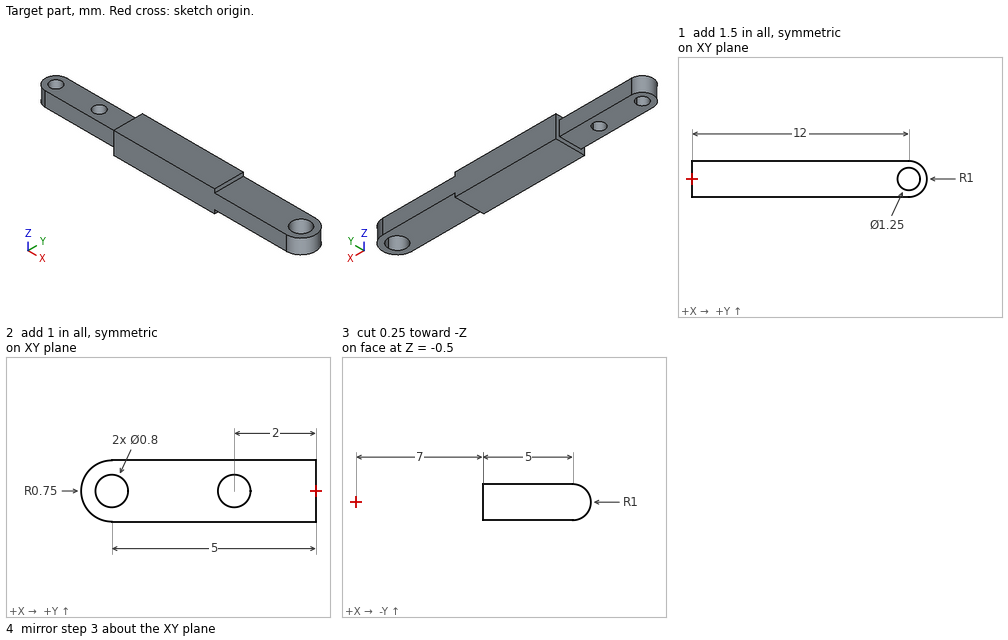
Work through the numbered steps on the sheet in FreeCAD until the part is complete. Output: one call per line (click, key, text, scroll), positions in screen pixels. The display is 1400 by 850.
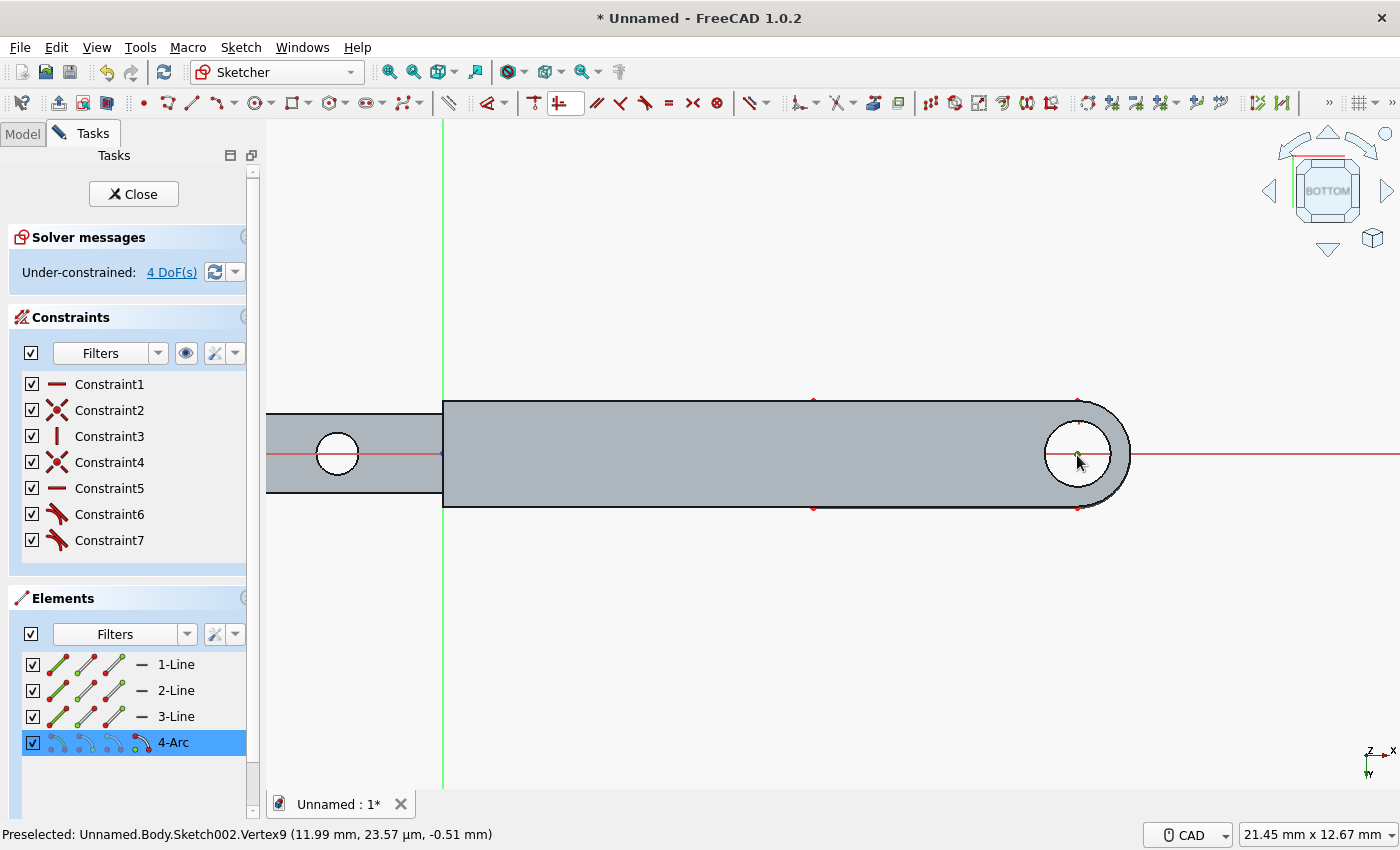
click(361, 454)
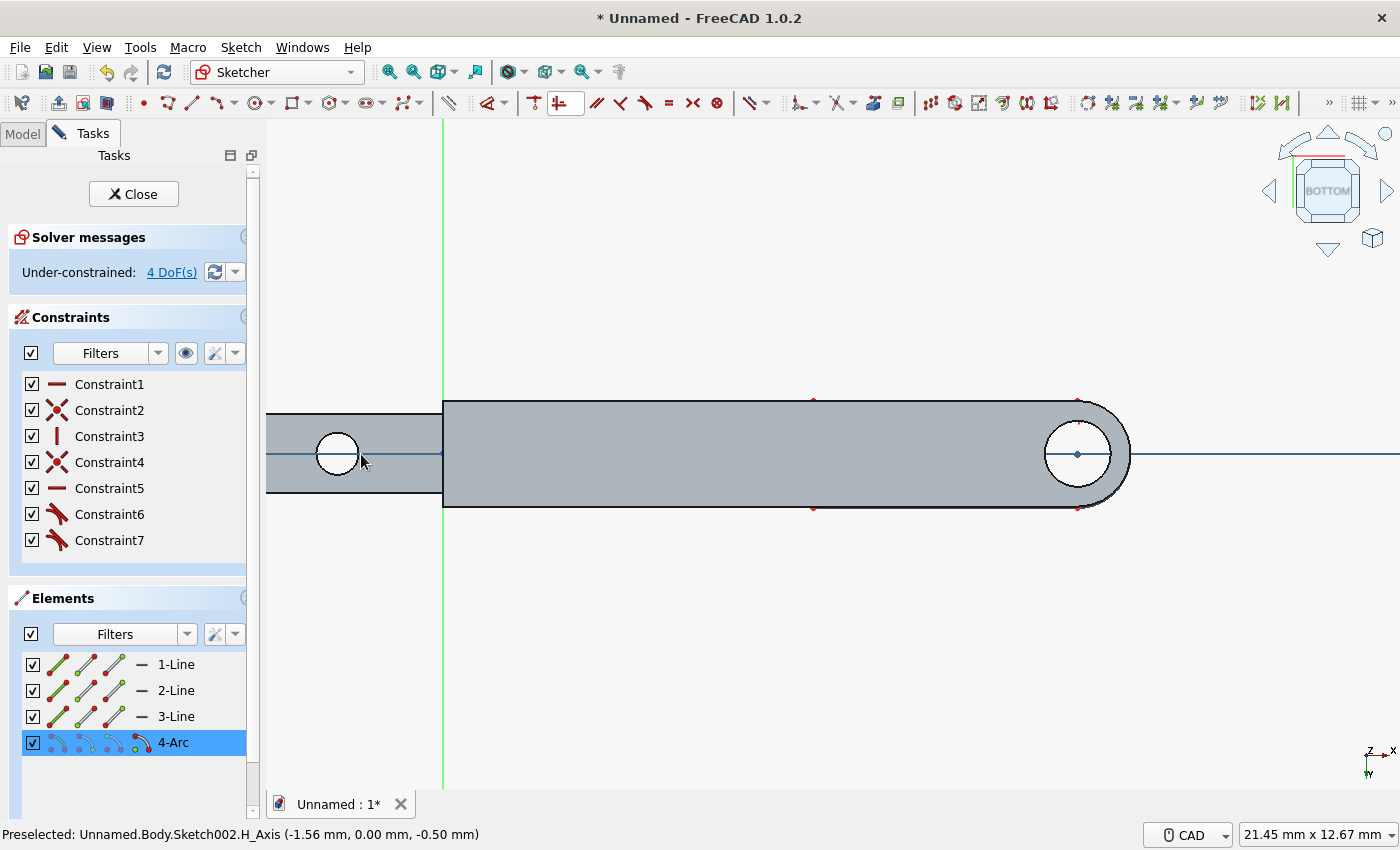
key(c)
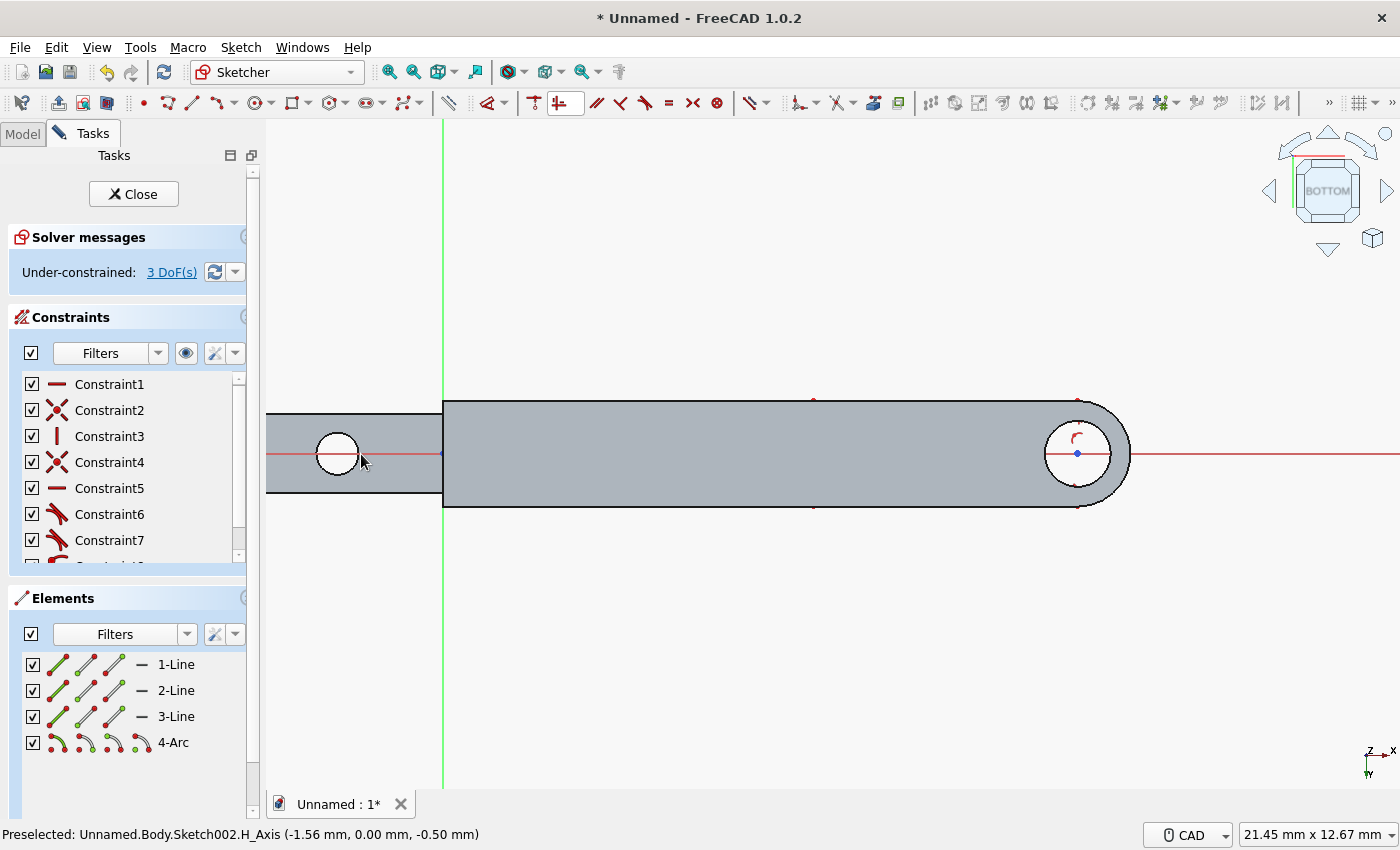
key(d)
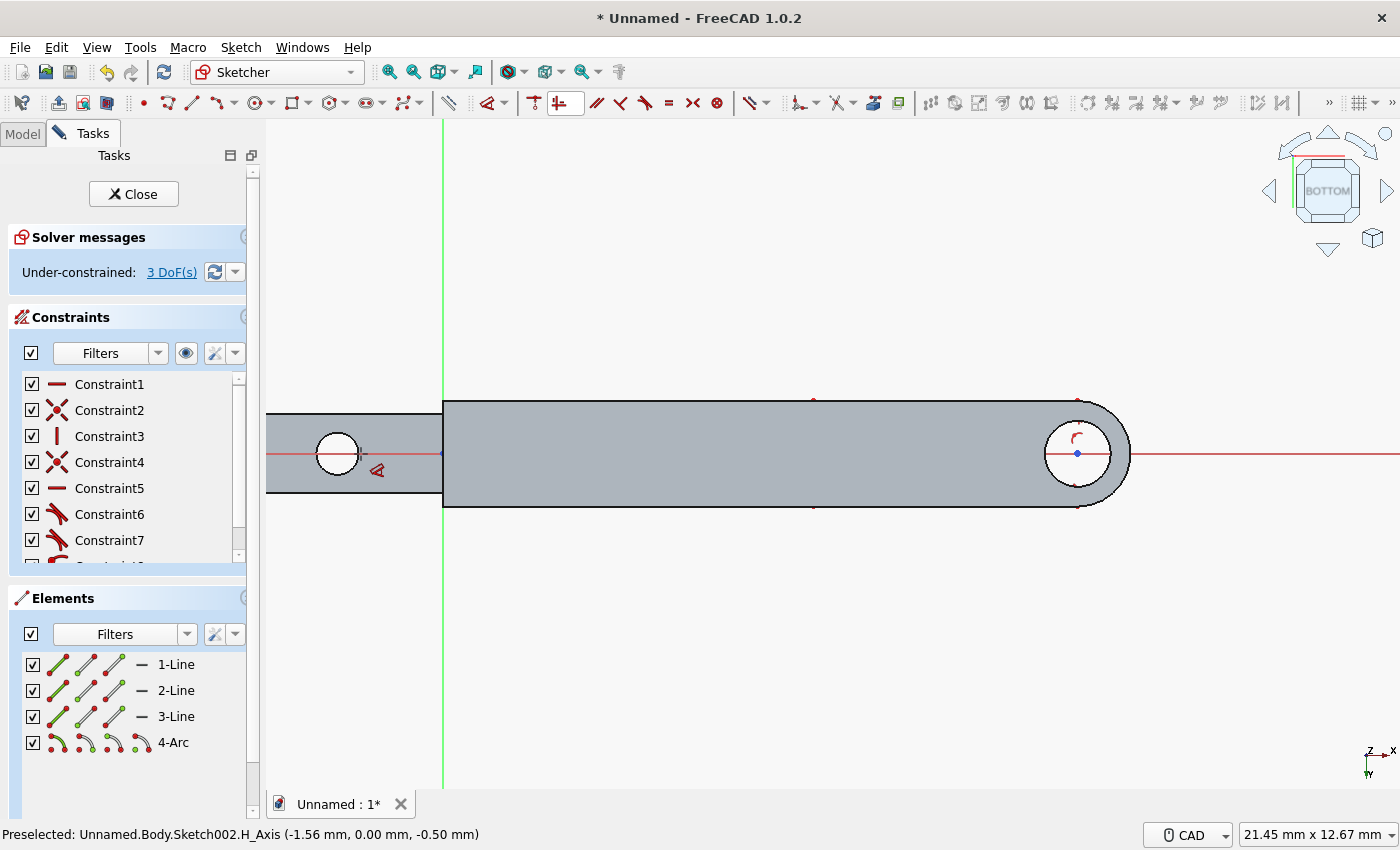
click(1119, 484)
click(1145, 503)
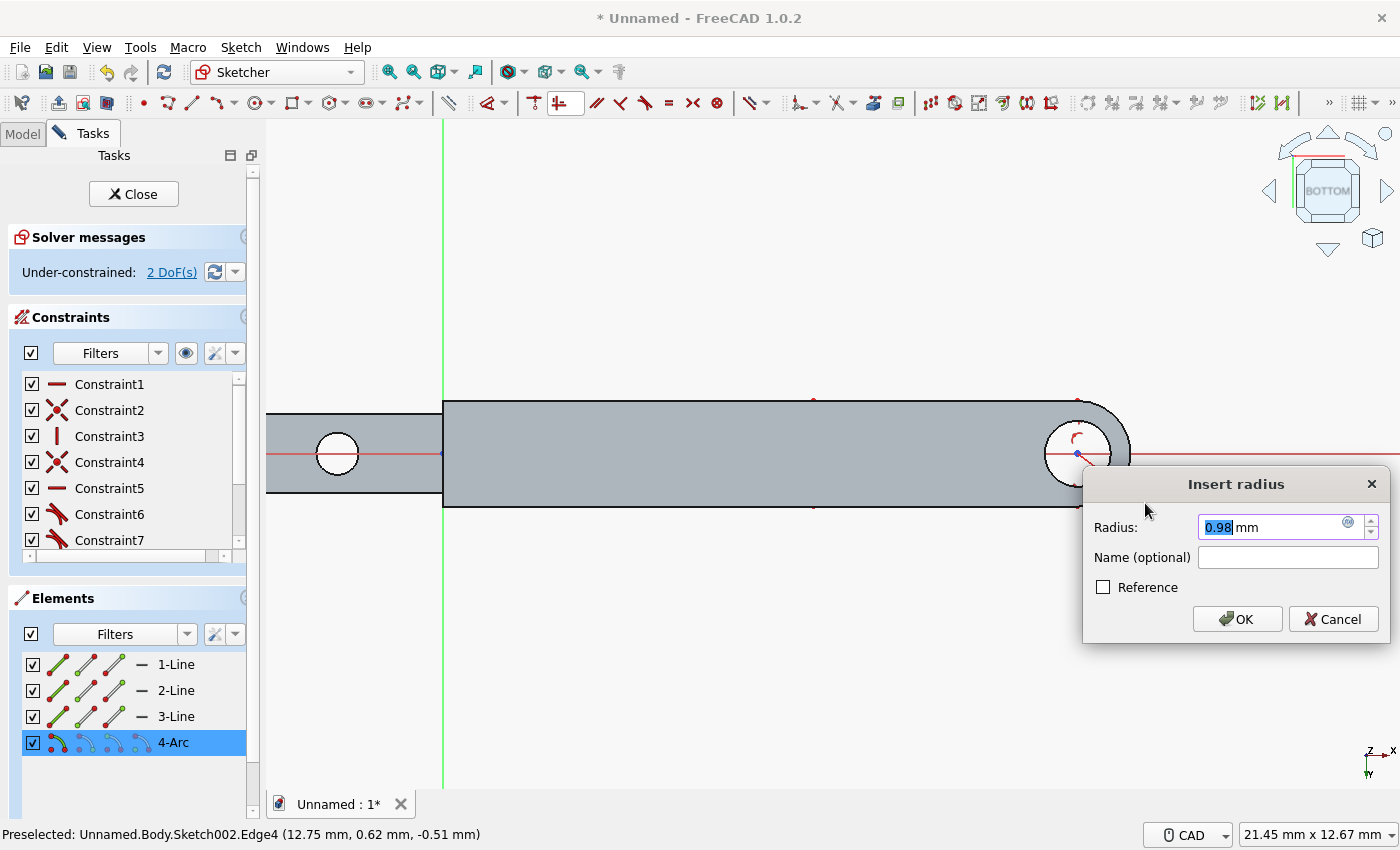
text(1)
key(Return)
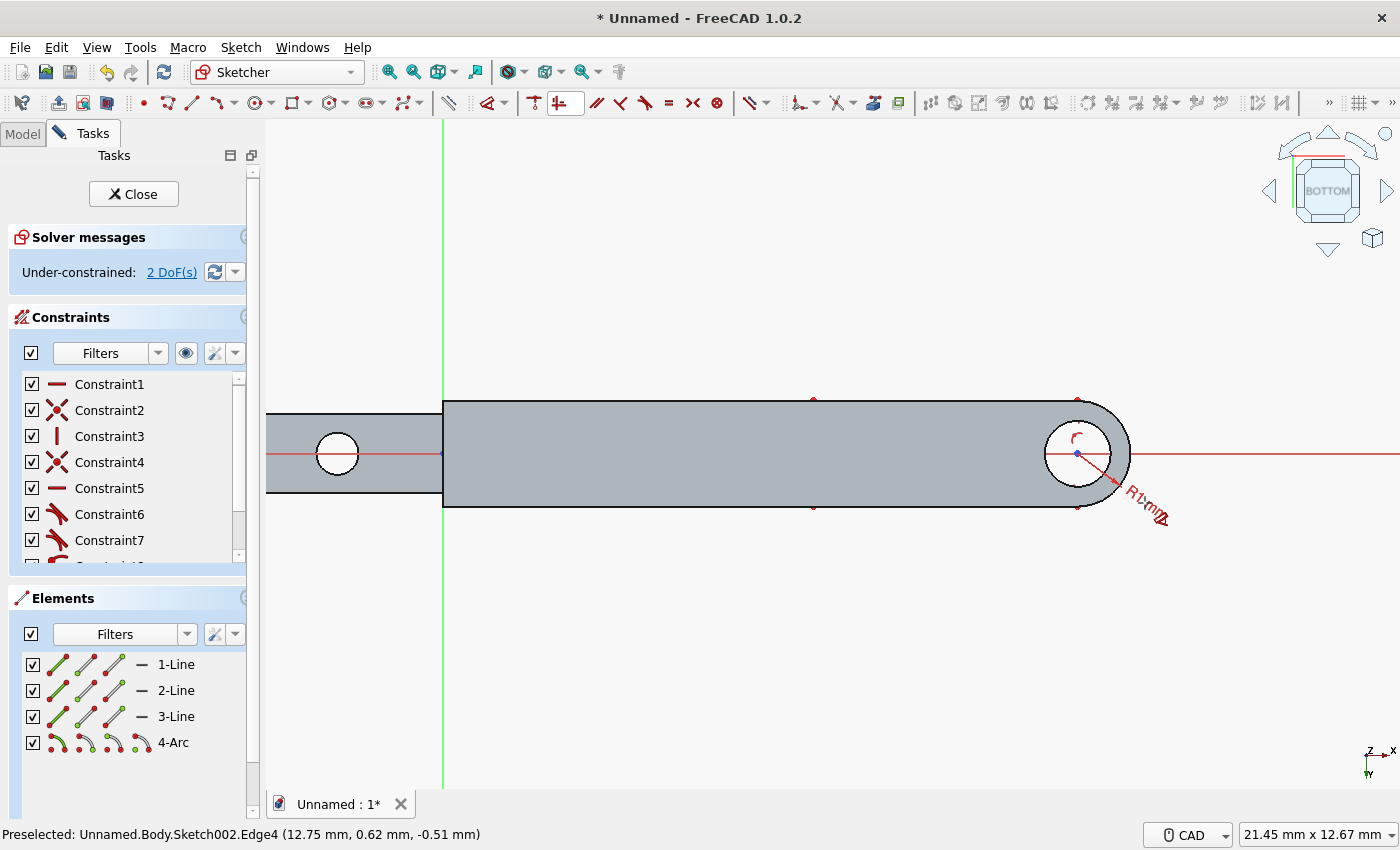
click(998, 401)
click(945, 367)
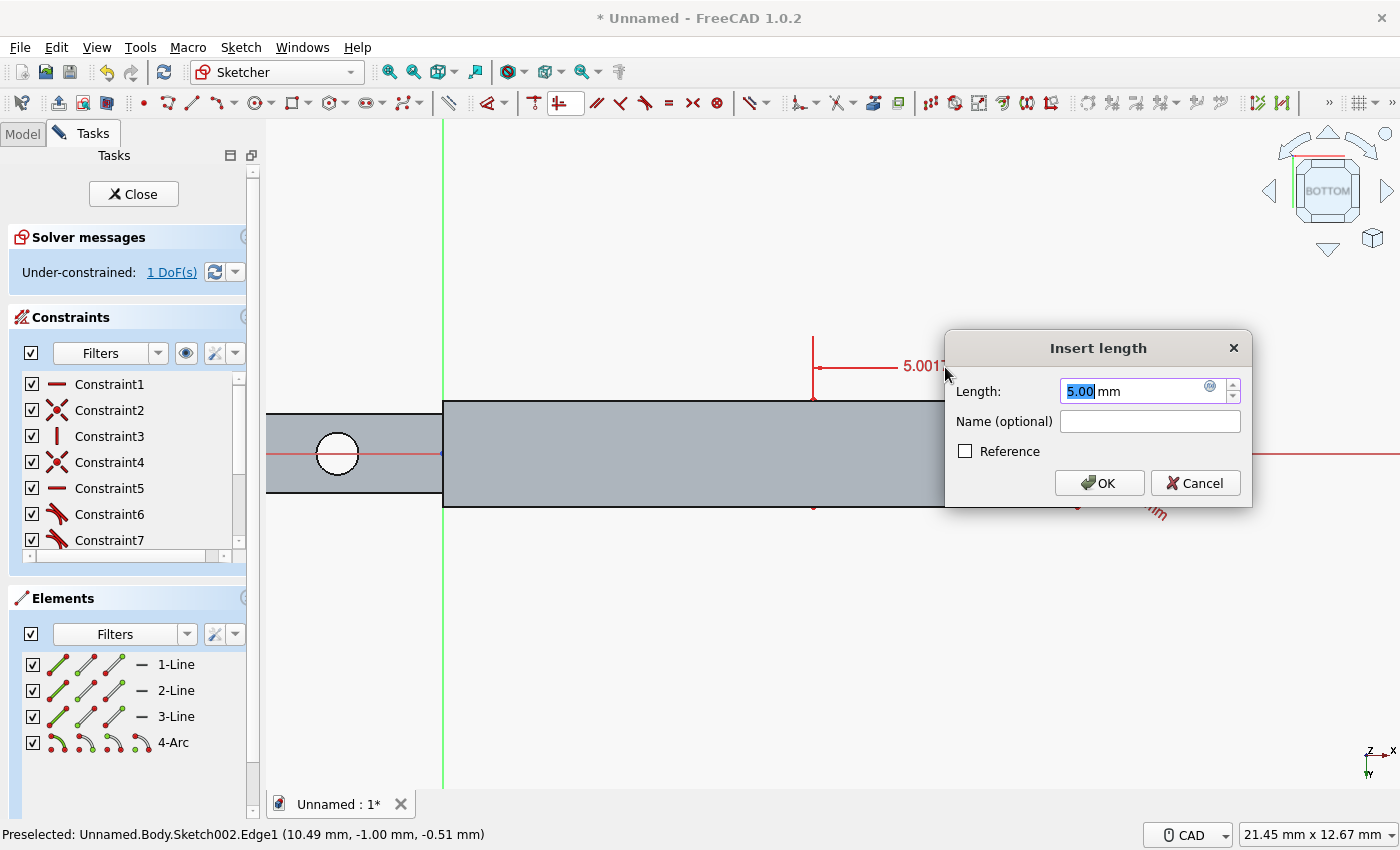
text(5)
key(Return)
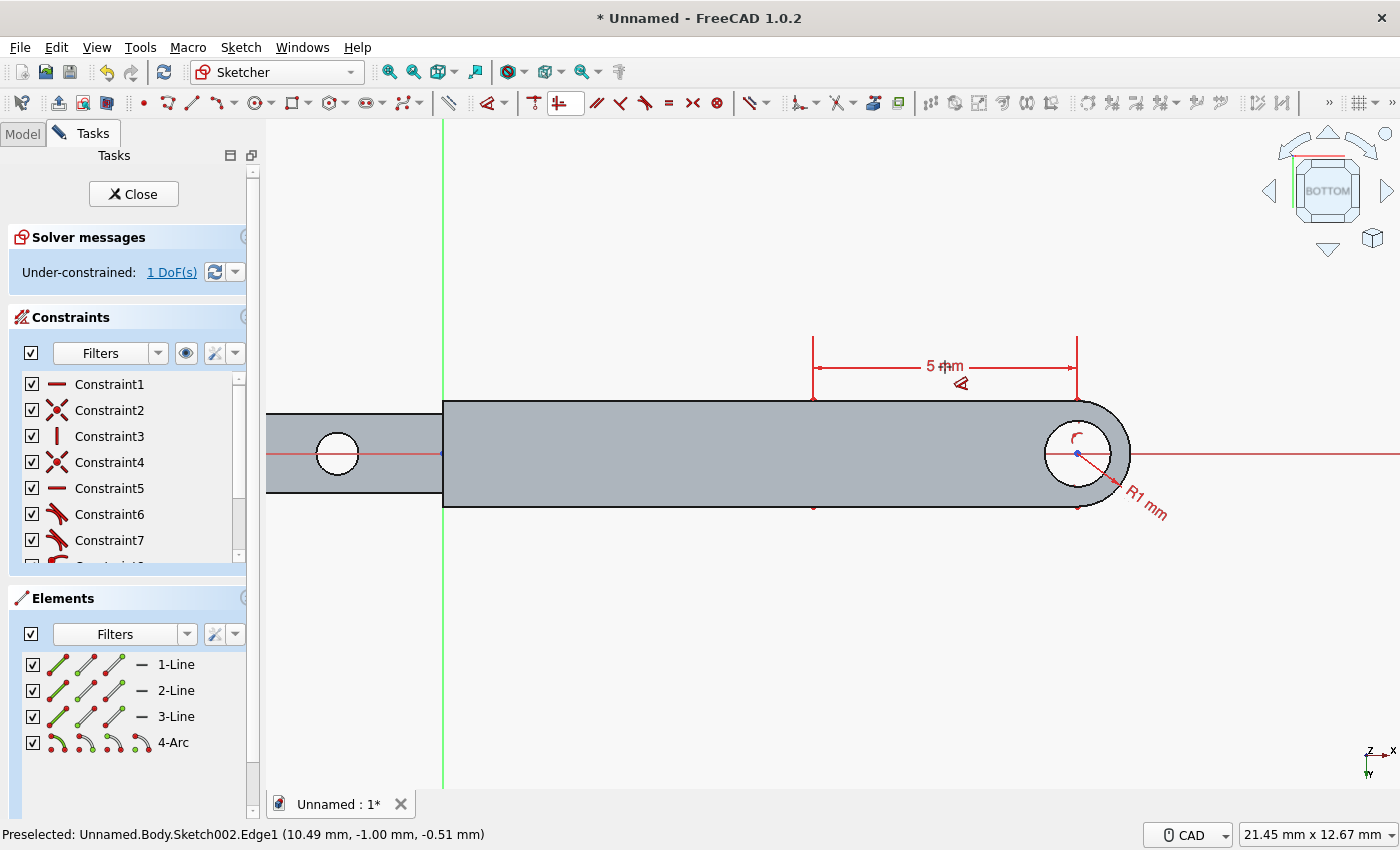
click(813, 401)
click(628, 367)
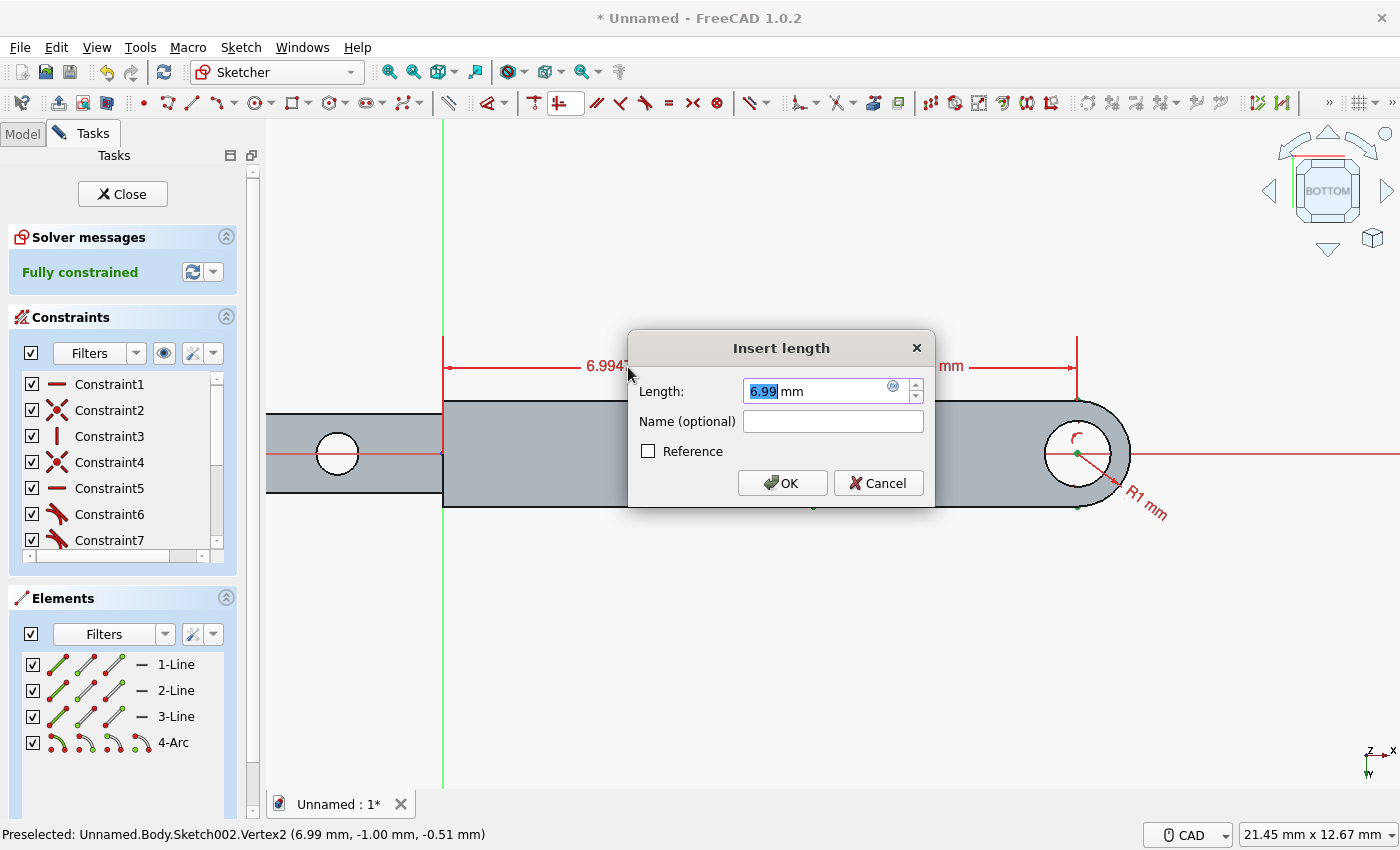
text(7)
key(Return)
key(Escape)